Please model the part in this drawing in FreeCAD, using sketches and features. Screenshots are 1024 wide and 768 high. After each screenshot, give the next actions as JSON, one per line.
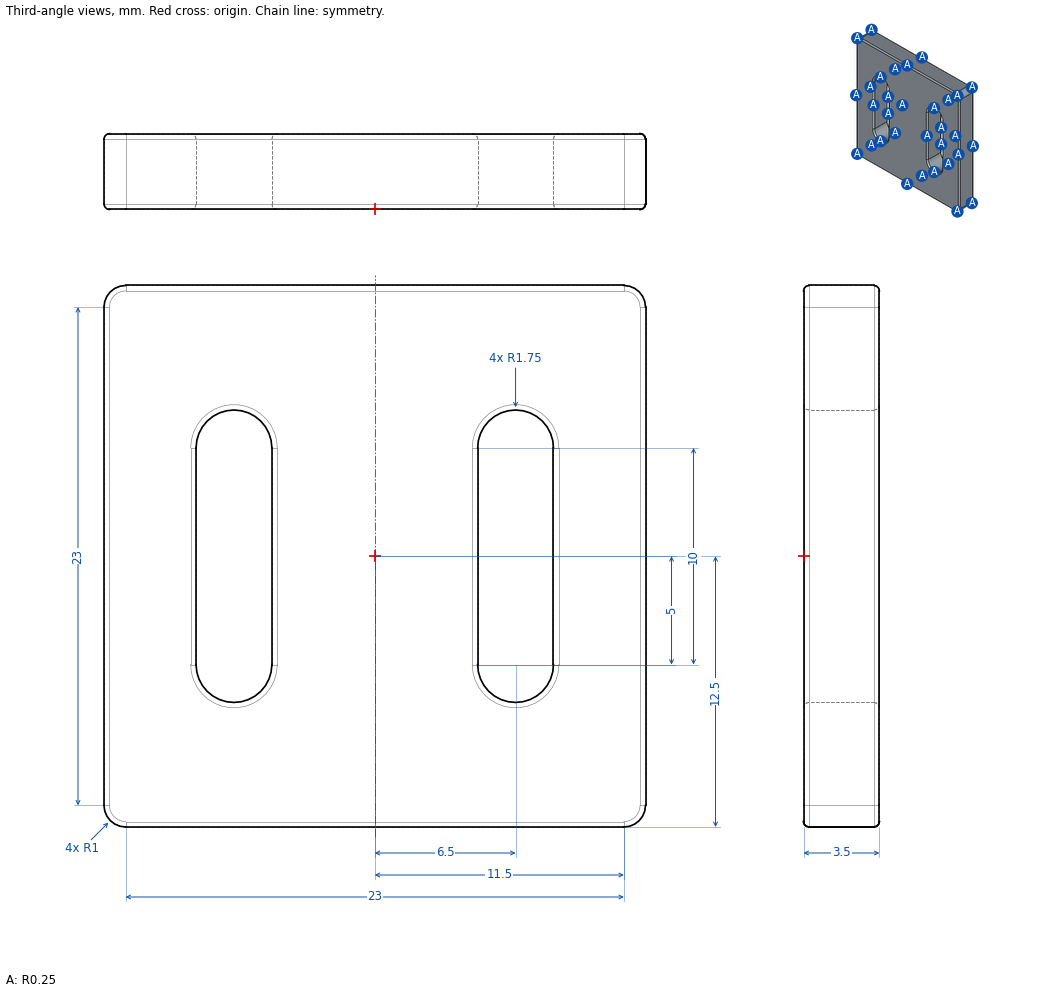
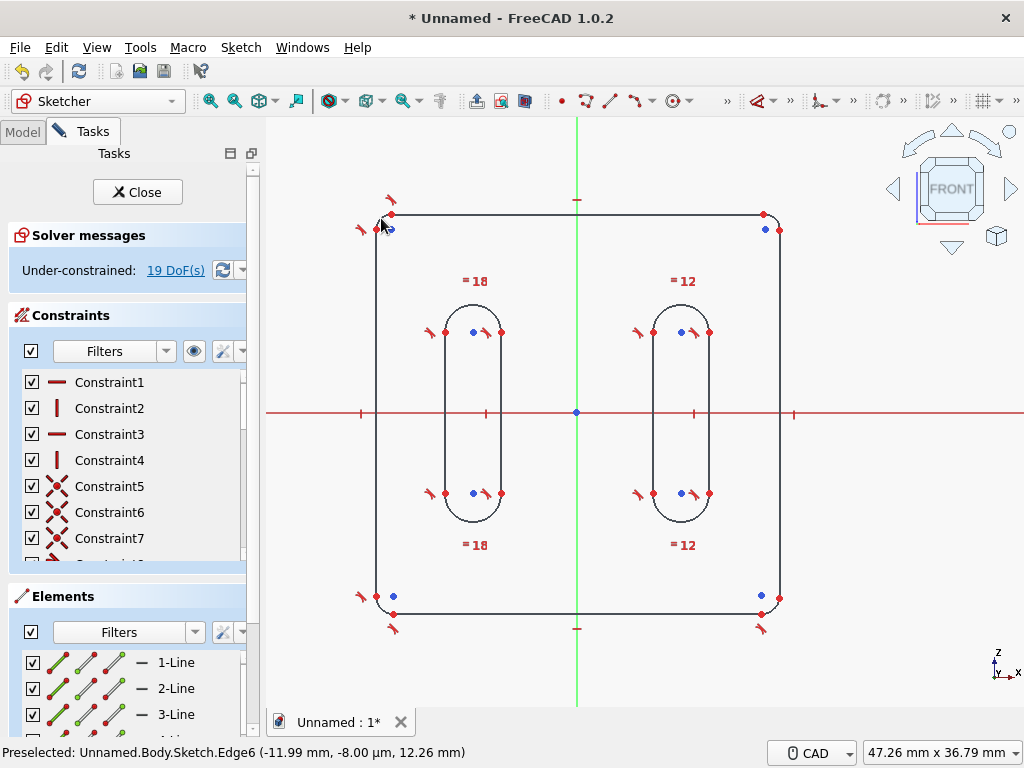
{"action": "left_click", "coordinate": [503, 215]}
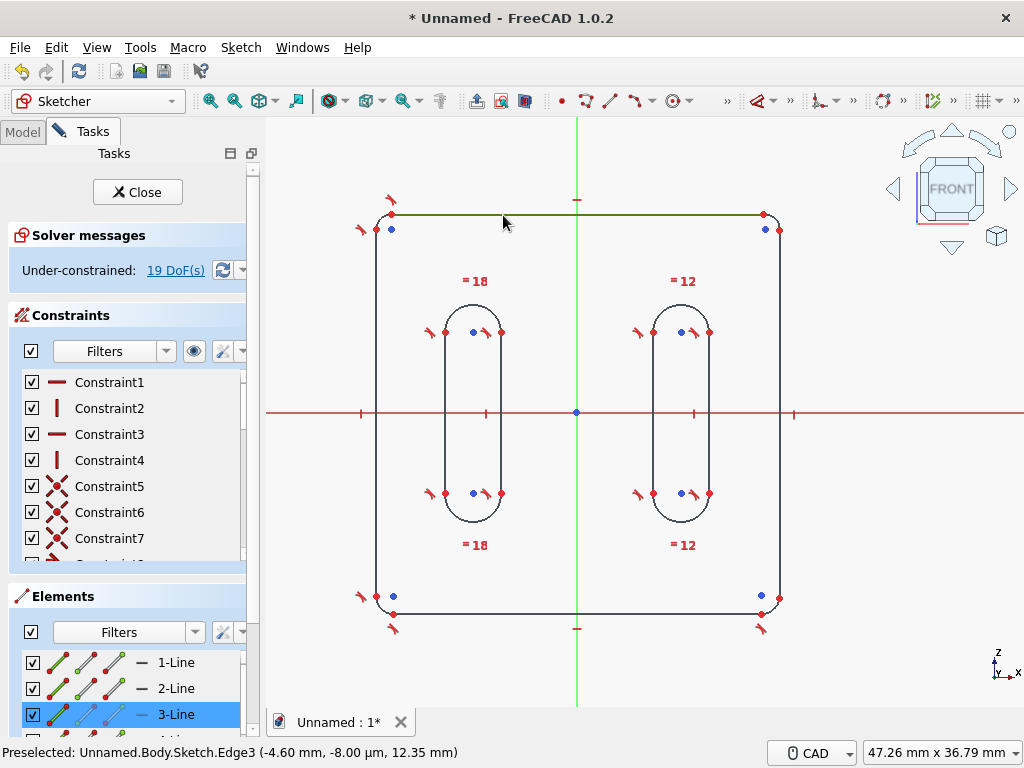
{"action": "left_click", "coordinate": [775, 219]}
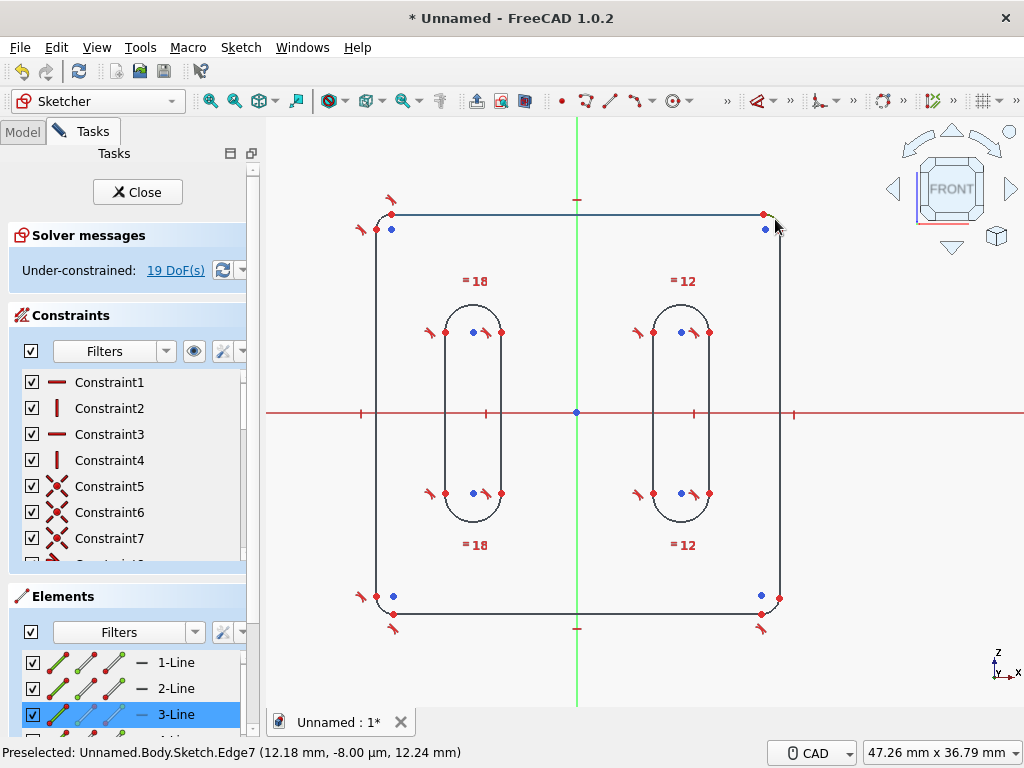
{"action": "key", "text": "t"}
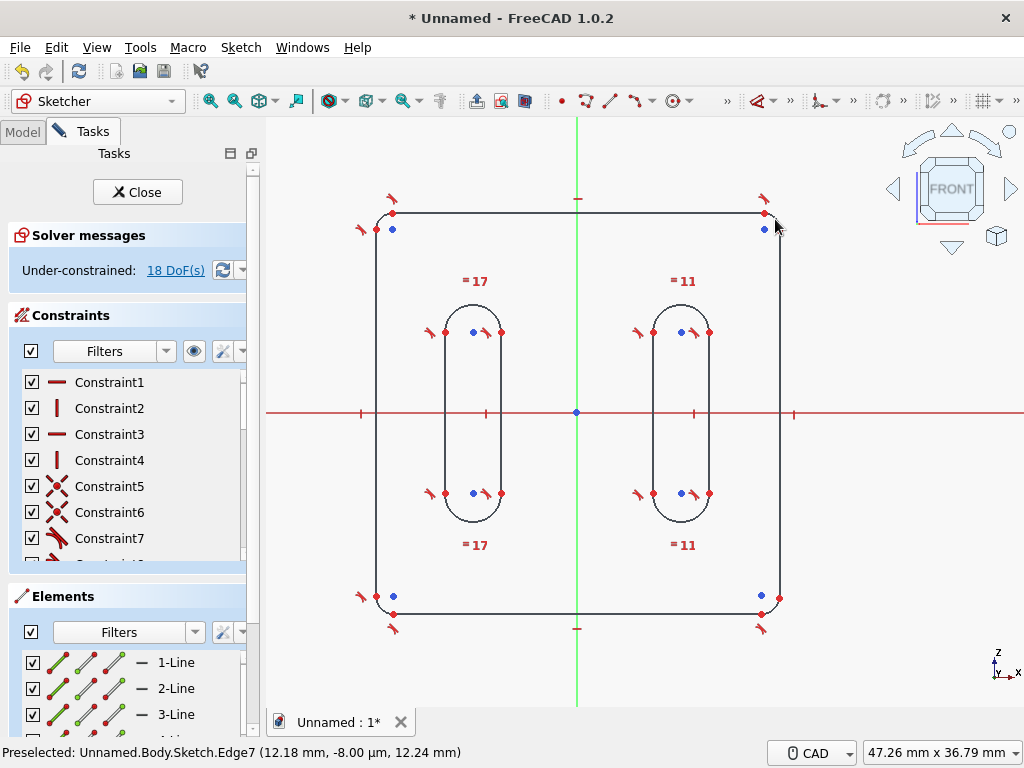
{"action": "left_click", "coordinate": [780, 341]}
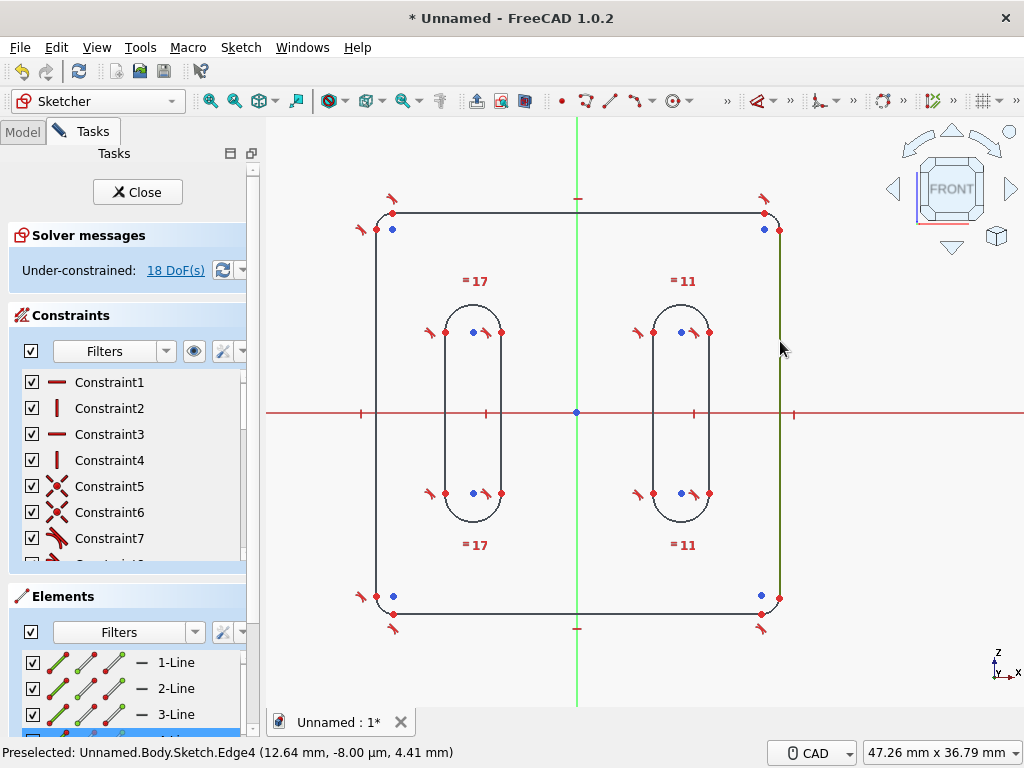
{"action": "left_click", "coordinate": [776, 219]}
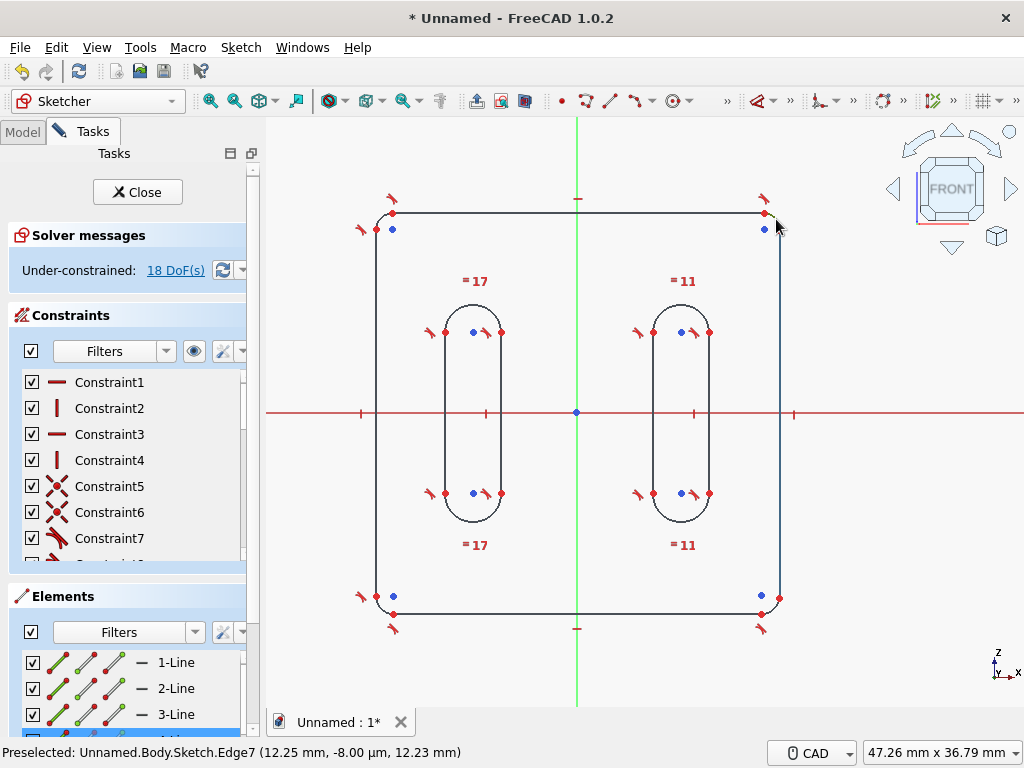
{"action": "key", "text": "t"}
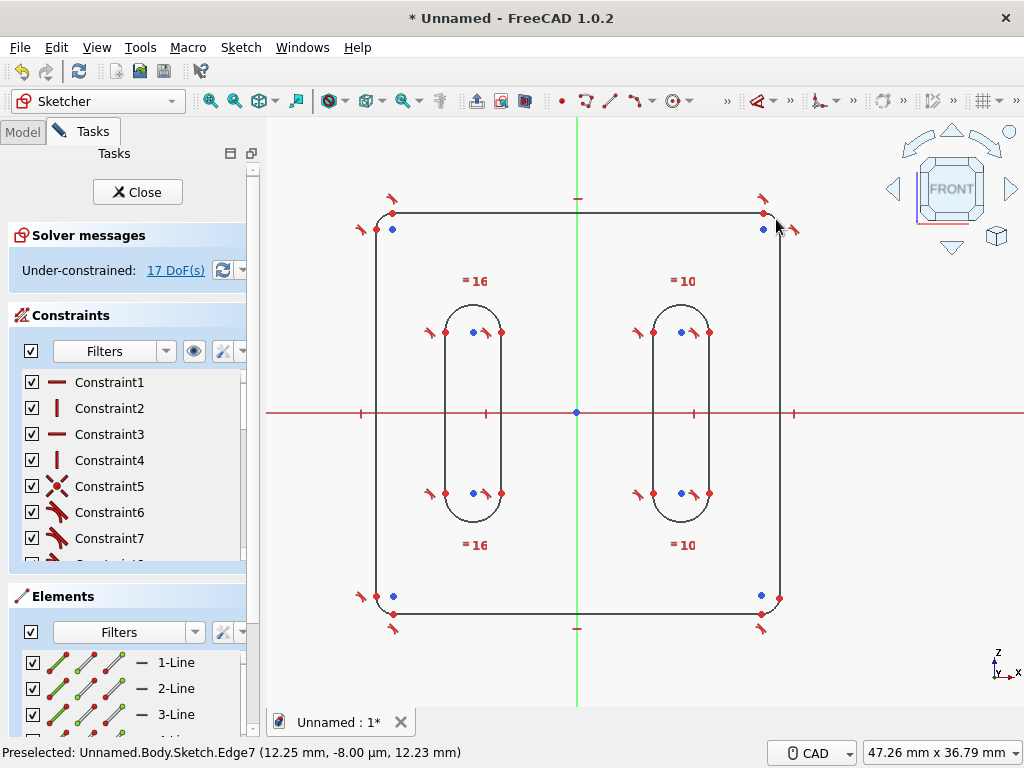
{"action": "left_click", "coordinate": [780, 340]}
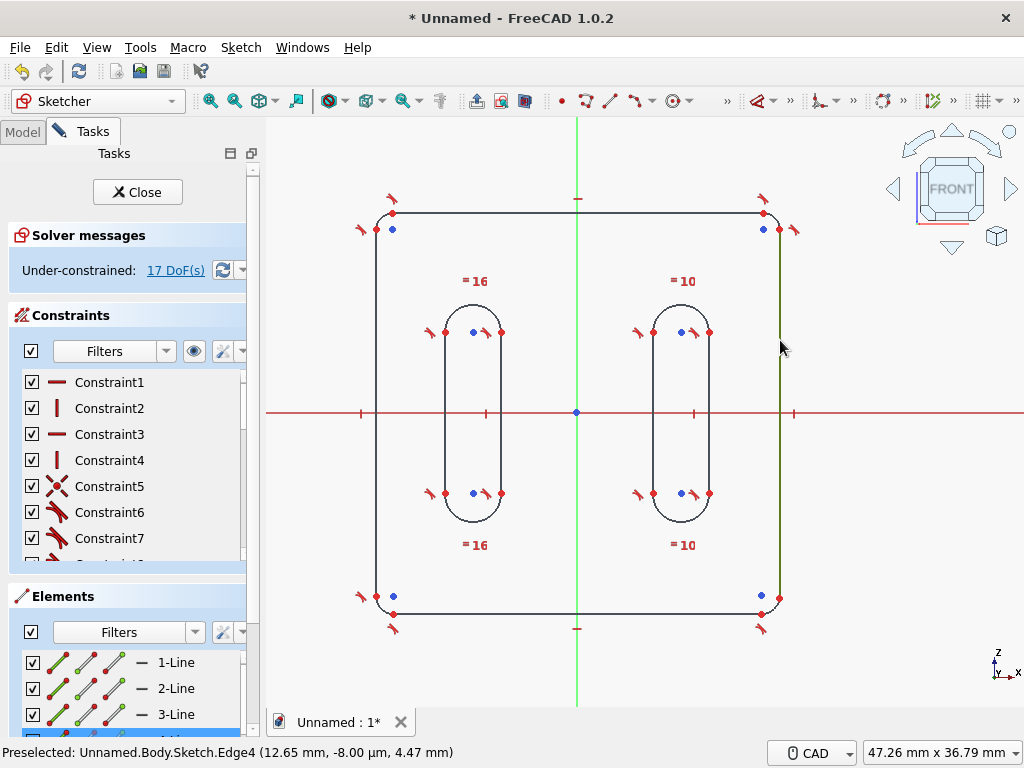
{"action": "left_click", "coordinate": [773, 610]}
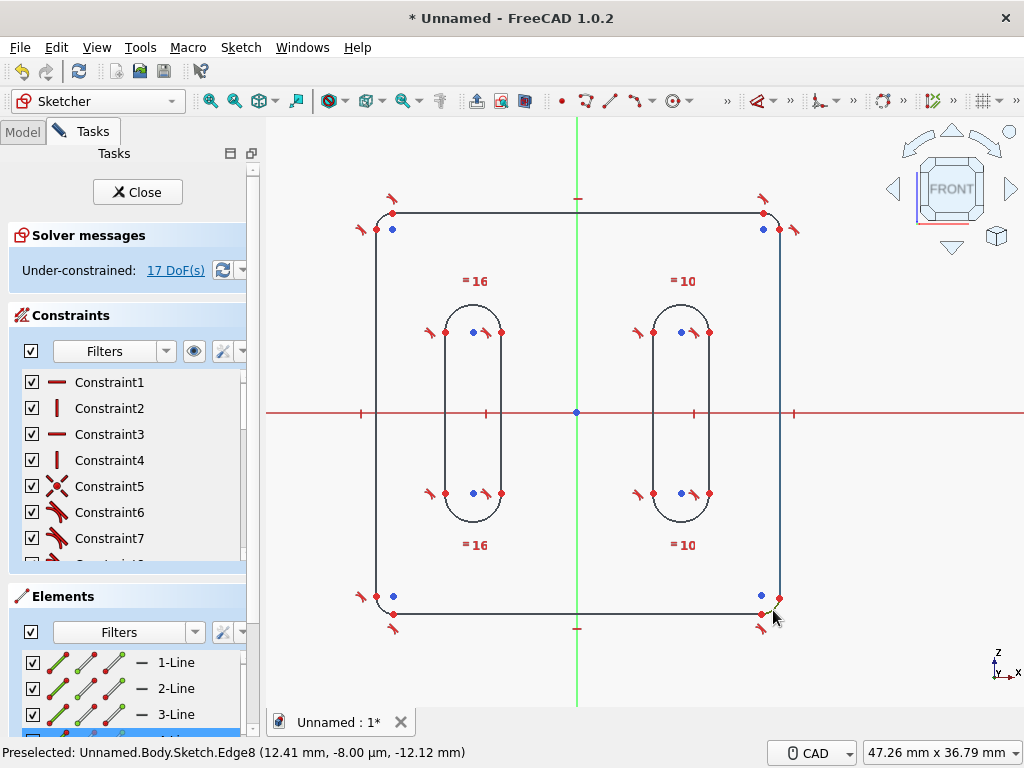
{"action": "key", "text": "t"}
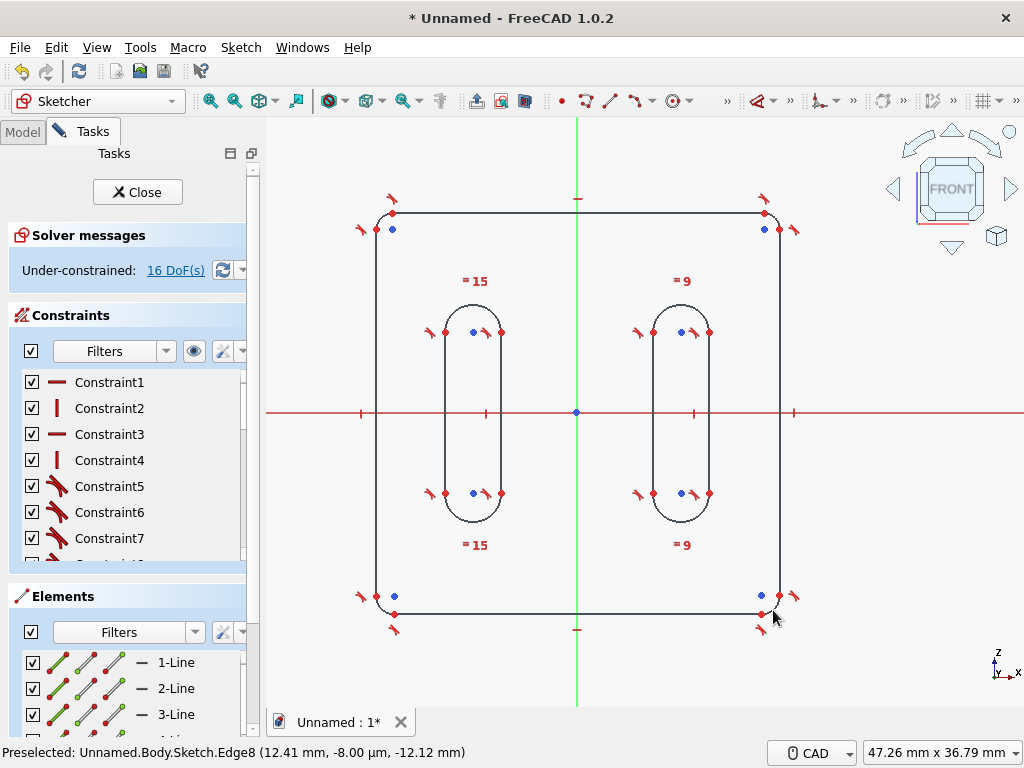
{"action": "left_click", "coordinate": [382, 609]}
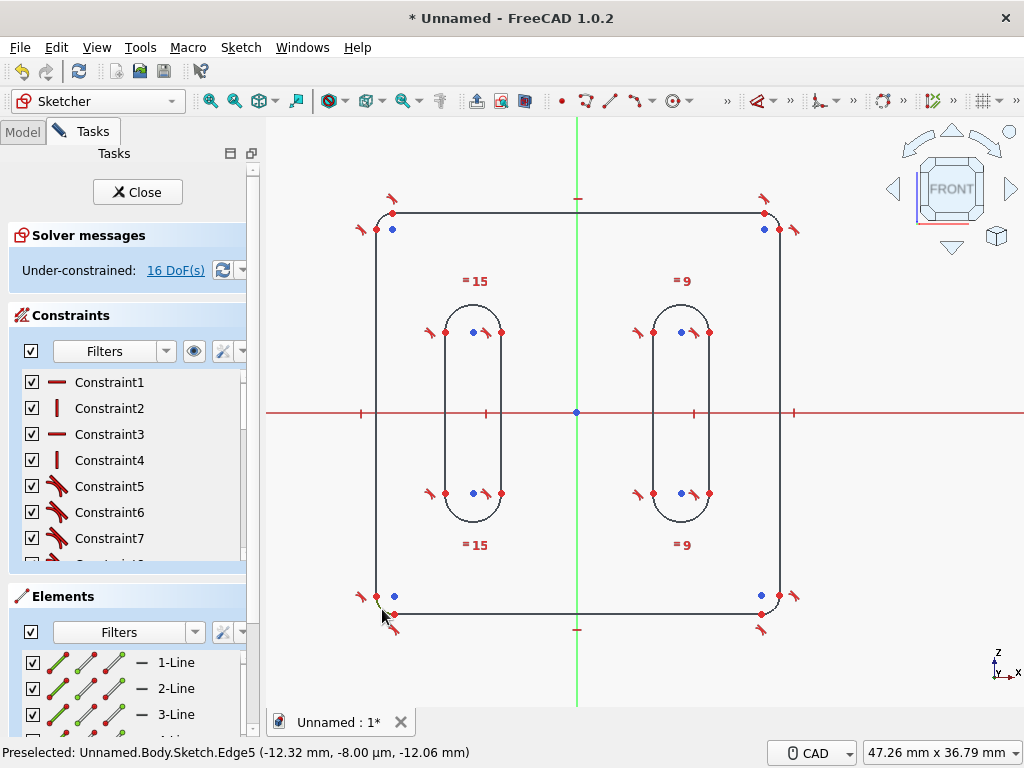
{"action": "left_click", "coordinate": [381, 218]}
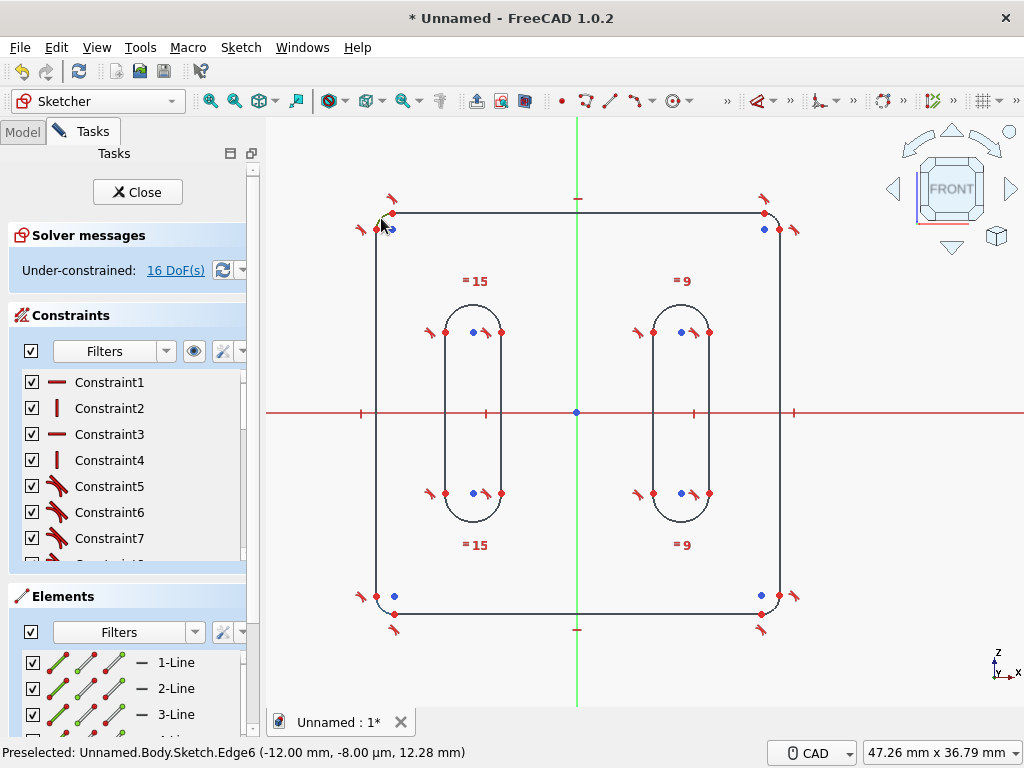
{"action": "left_click", "coordinate": [775, 218]}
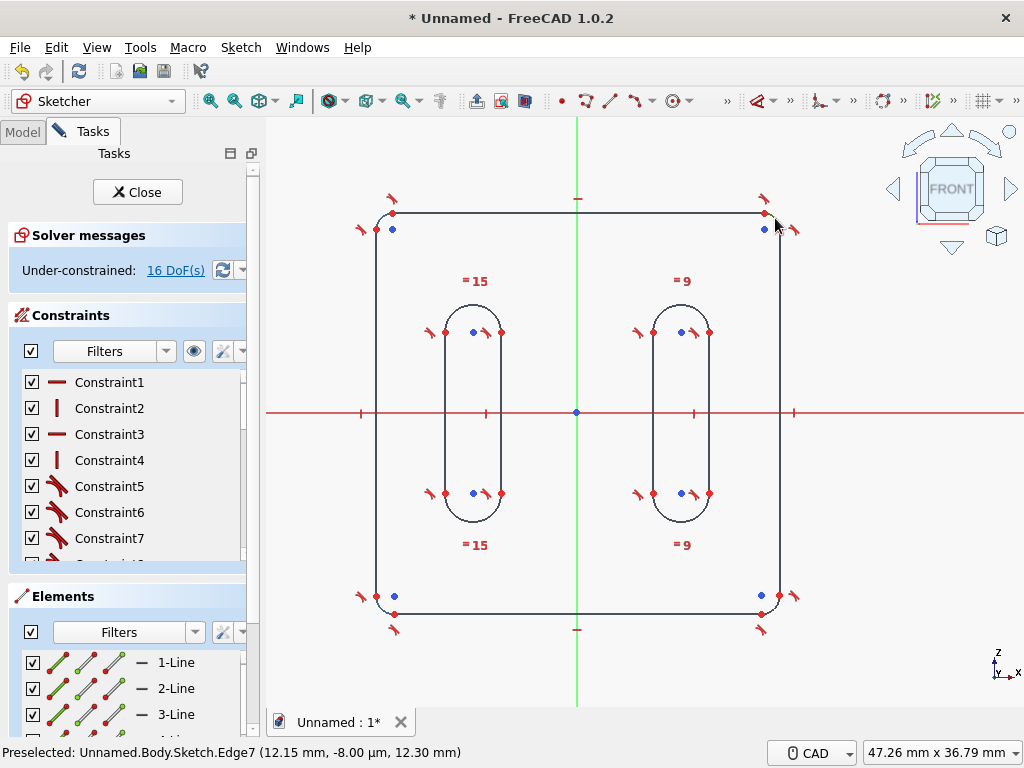
{"action": "left_click", "coordinate": [774, 609]}